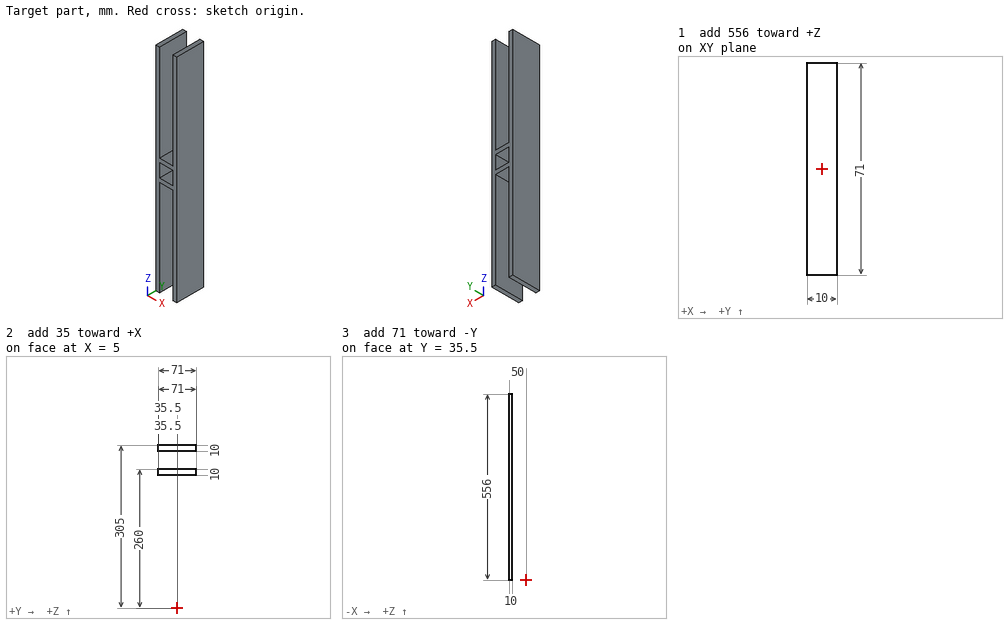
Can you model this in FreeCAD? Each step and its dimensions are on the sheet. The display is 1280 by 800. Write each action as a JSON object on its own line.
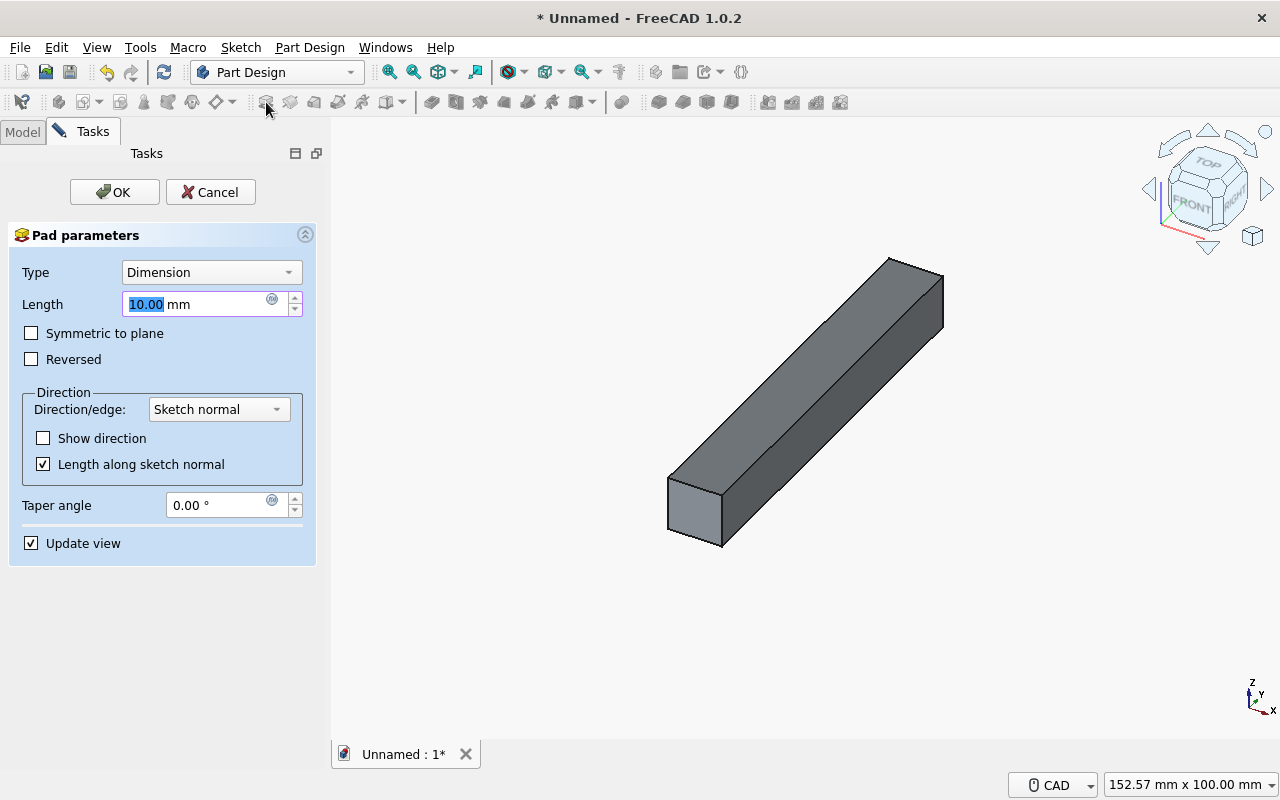
{"action": "type", "text": "556"}
{"action": "key", "text": "Tab"}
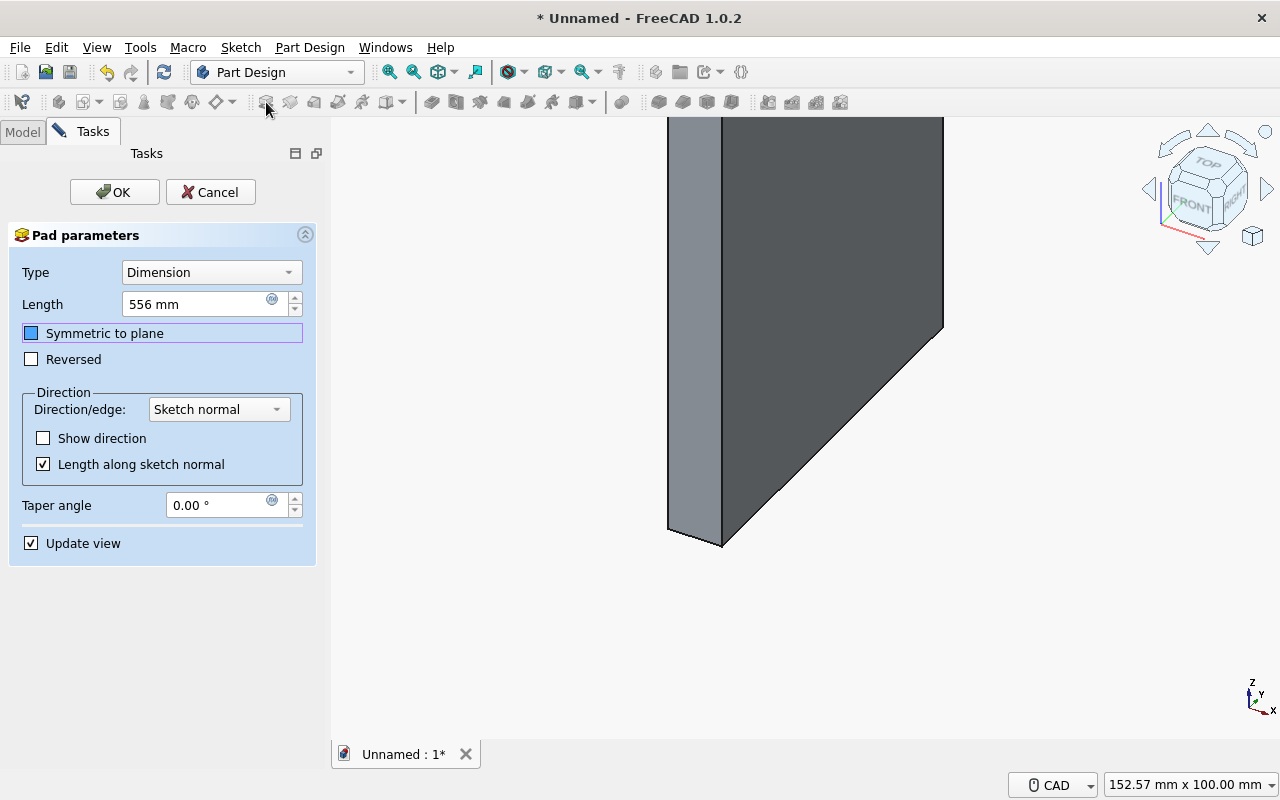
{"action": "left_click", "coordinate": [115, 192]}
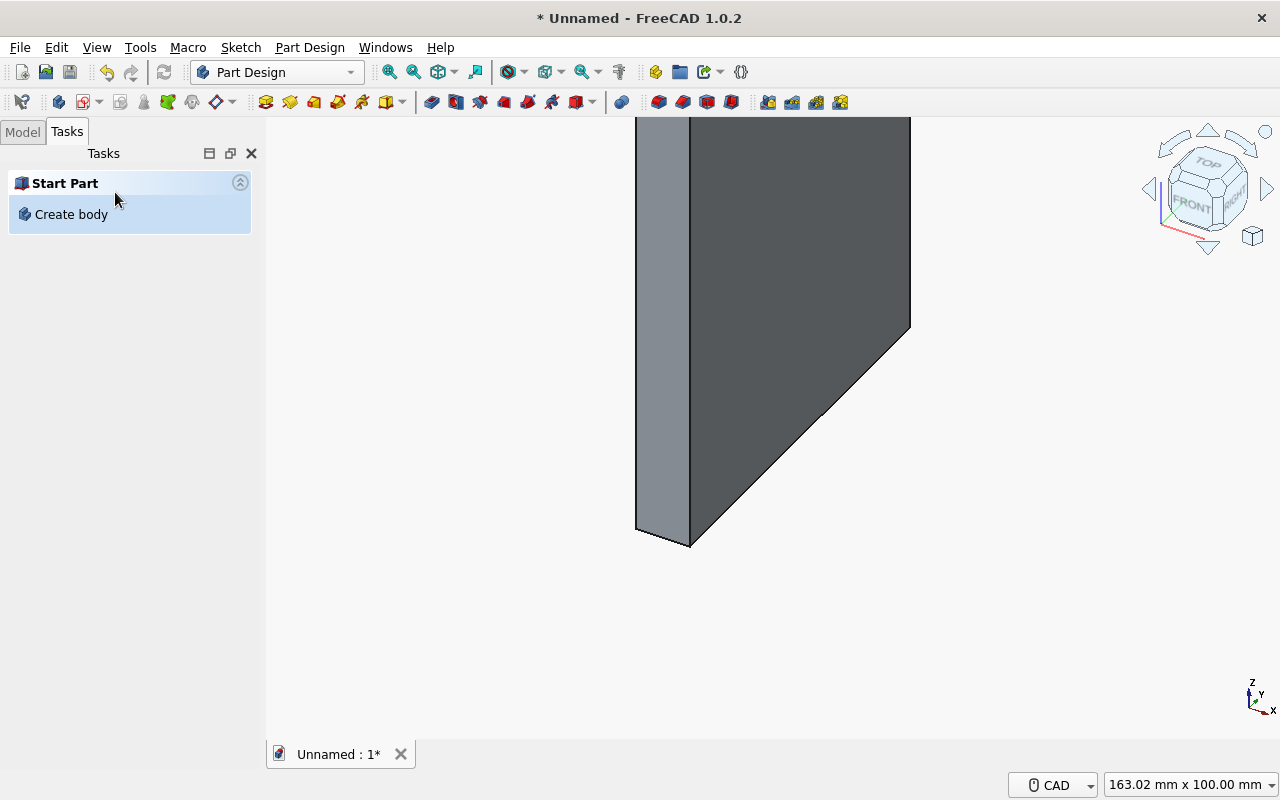
{"action": "left_click", "coordinate": [390, 72]}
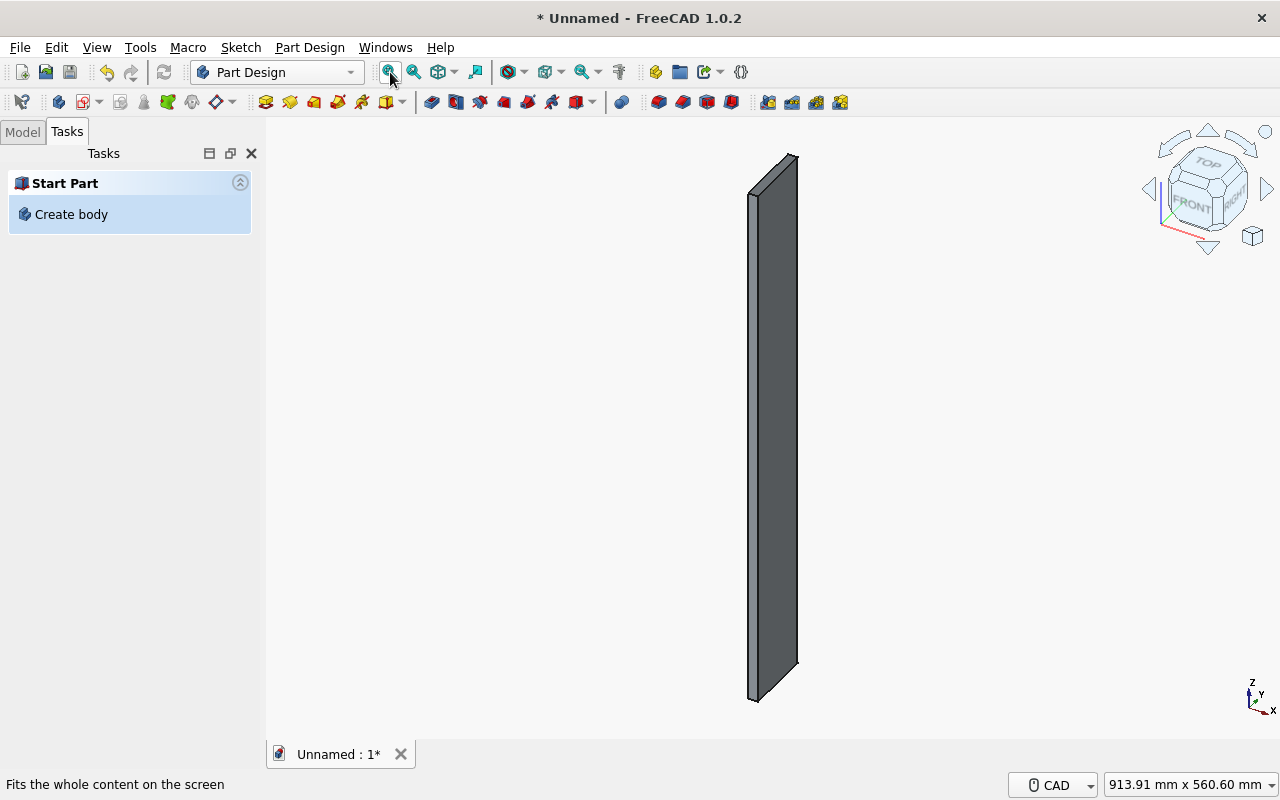
{"action": "left_click", "coordinate": [778, 212]}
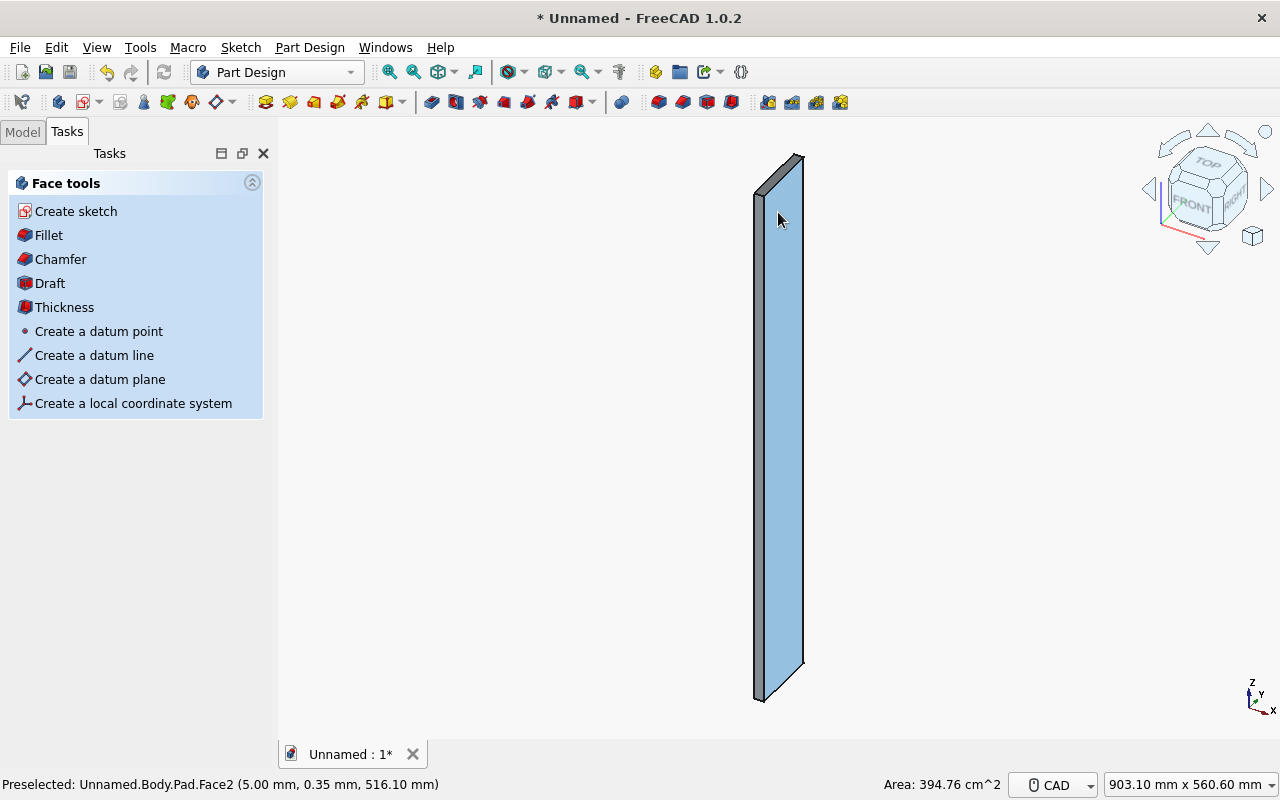
{"action": "left_click", "coordinate": [84, 102]}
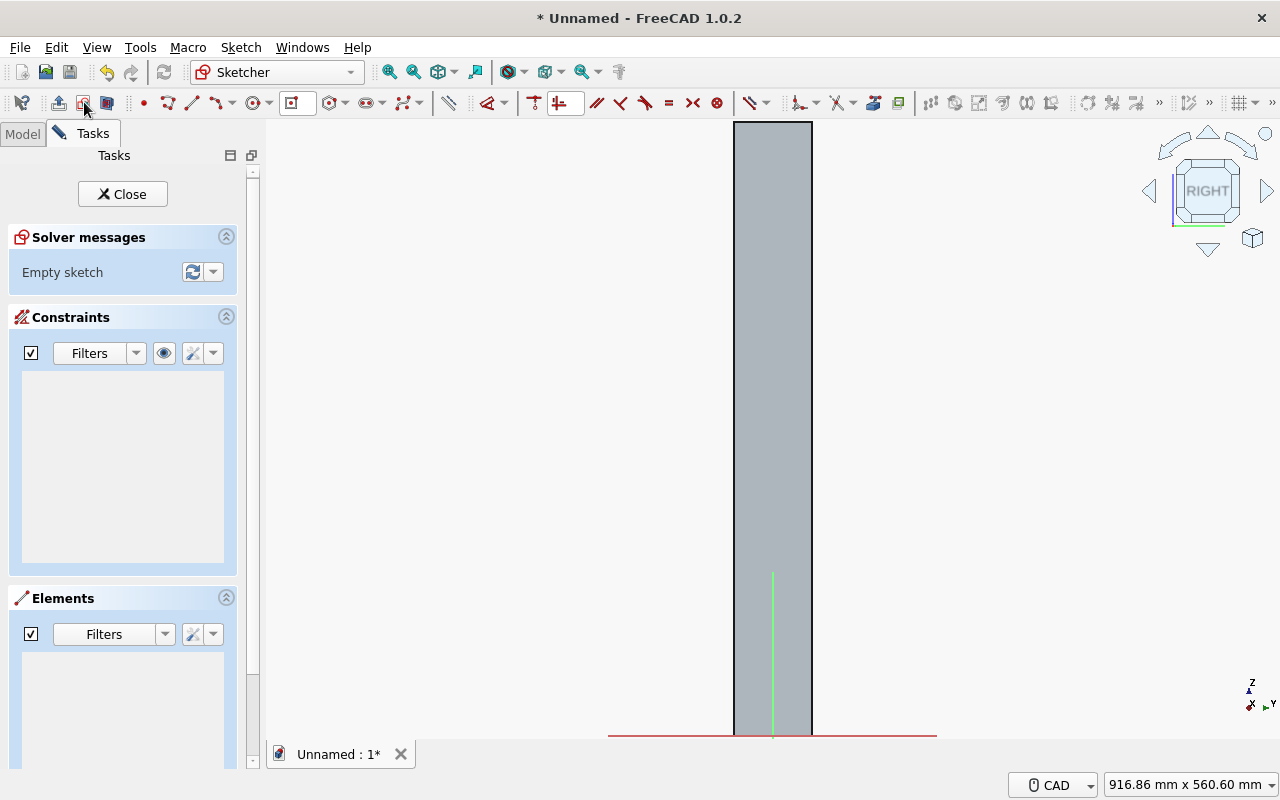
{"action": "scroll", "coordinate": [787, 430], "scroll_direction": "up", "scroll_amount": 9}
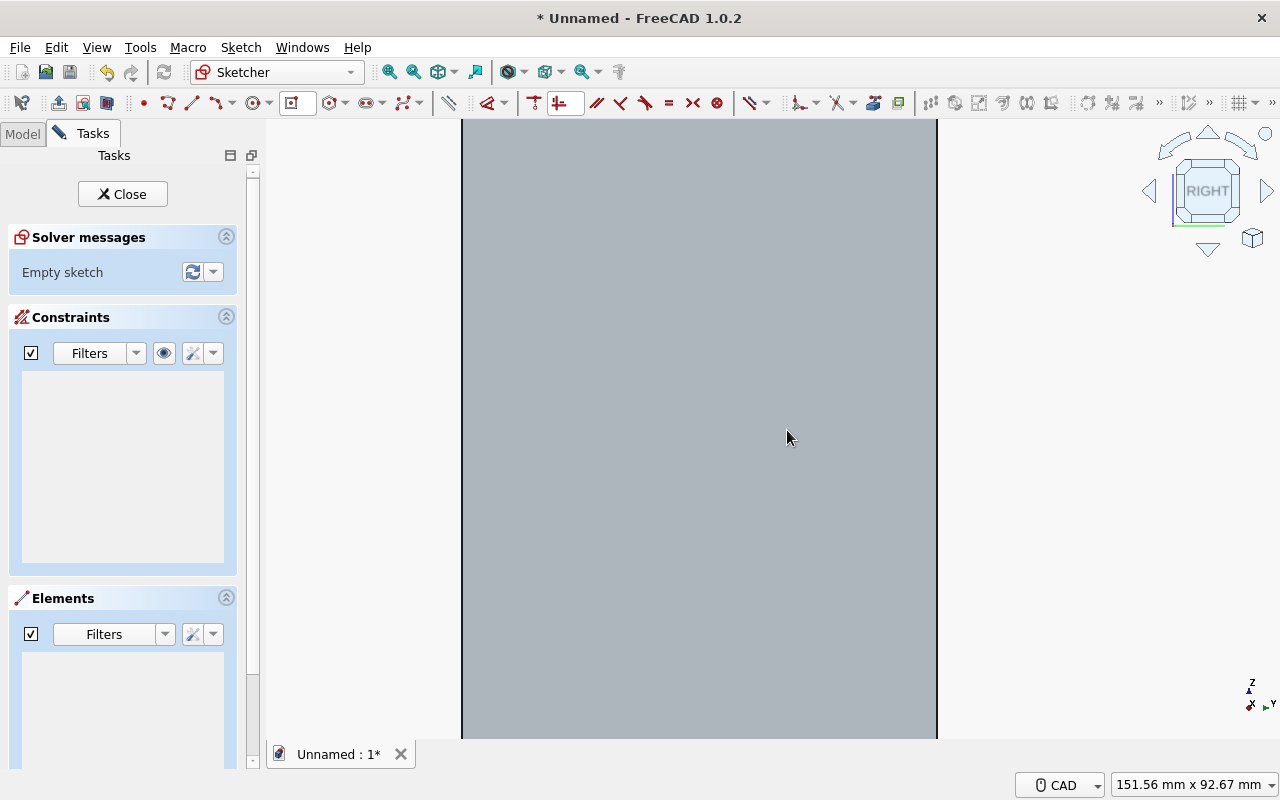
{"action": "key", "text": "g r"}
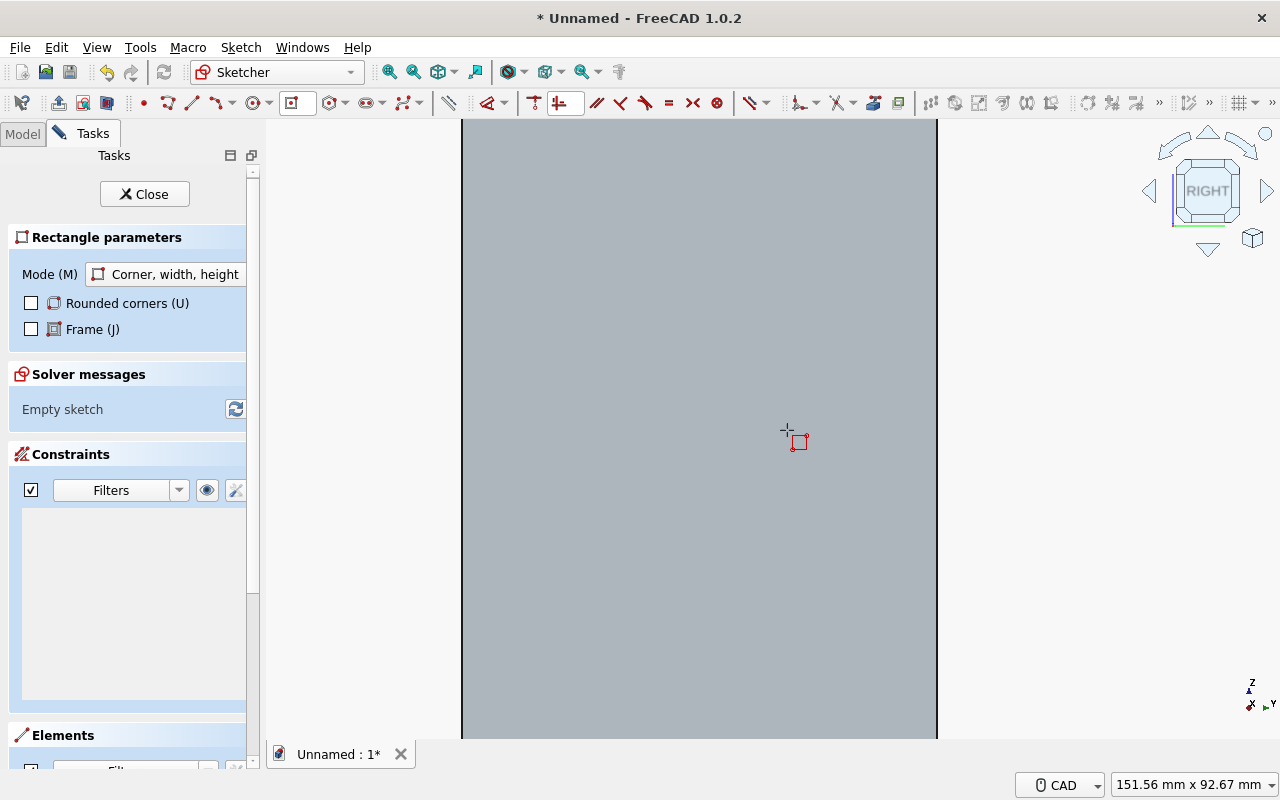
{"action": "left_click", "coordinate": [462, 241]}
{"action": "mouse_move", "coordinate": [937, 308]}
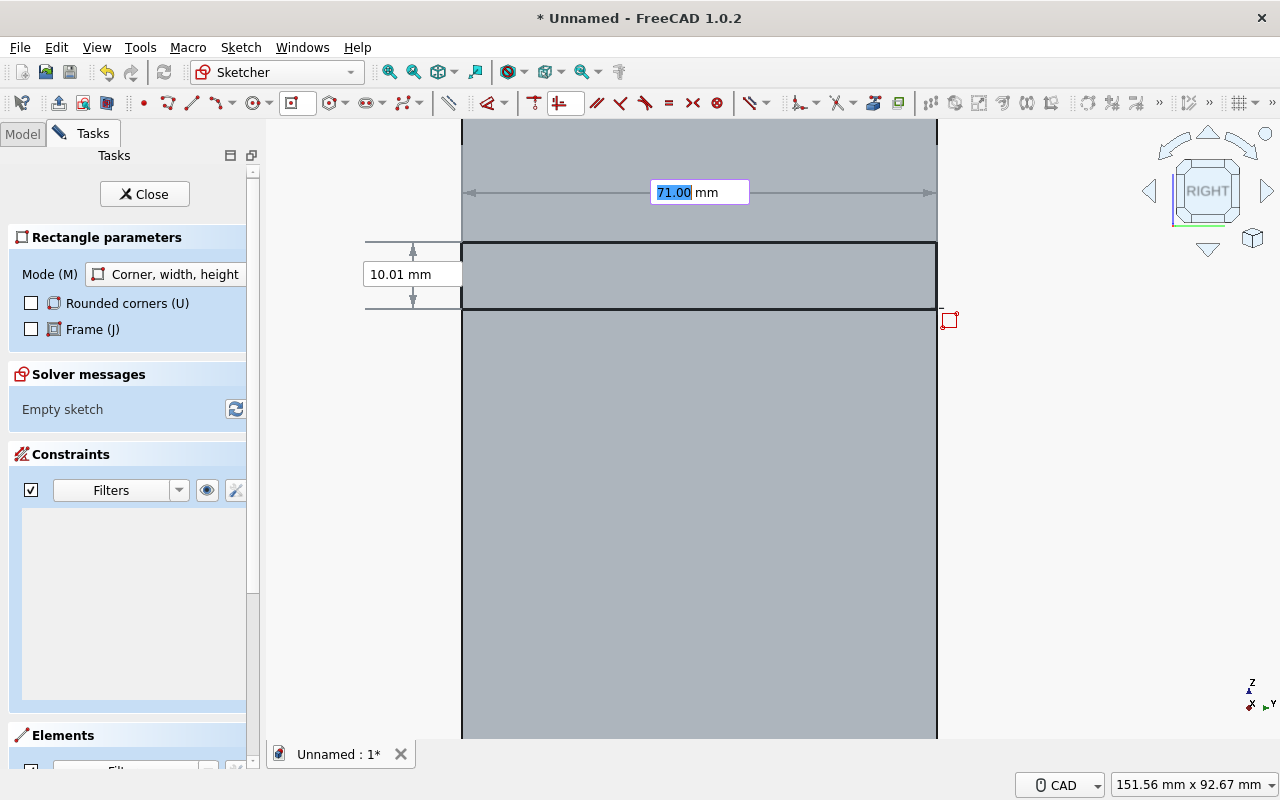
{"action": "type", "text": "71"}
{"action": "key", "text": "Tab"}
{"action": "type", "text": "10"}
{"action": "key", "text": "Return"}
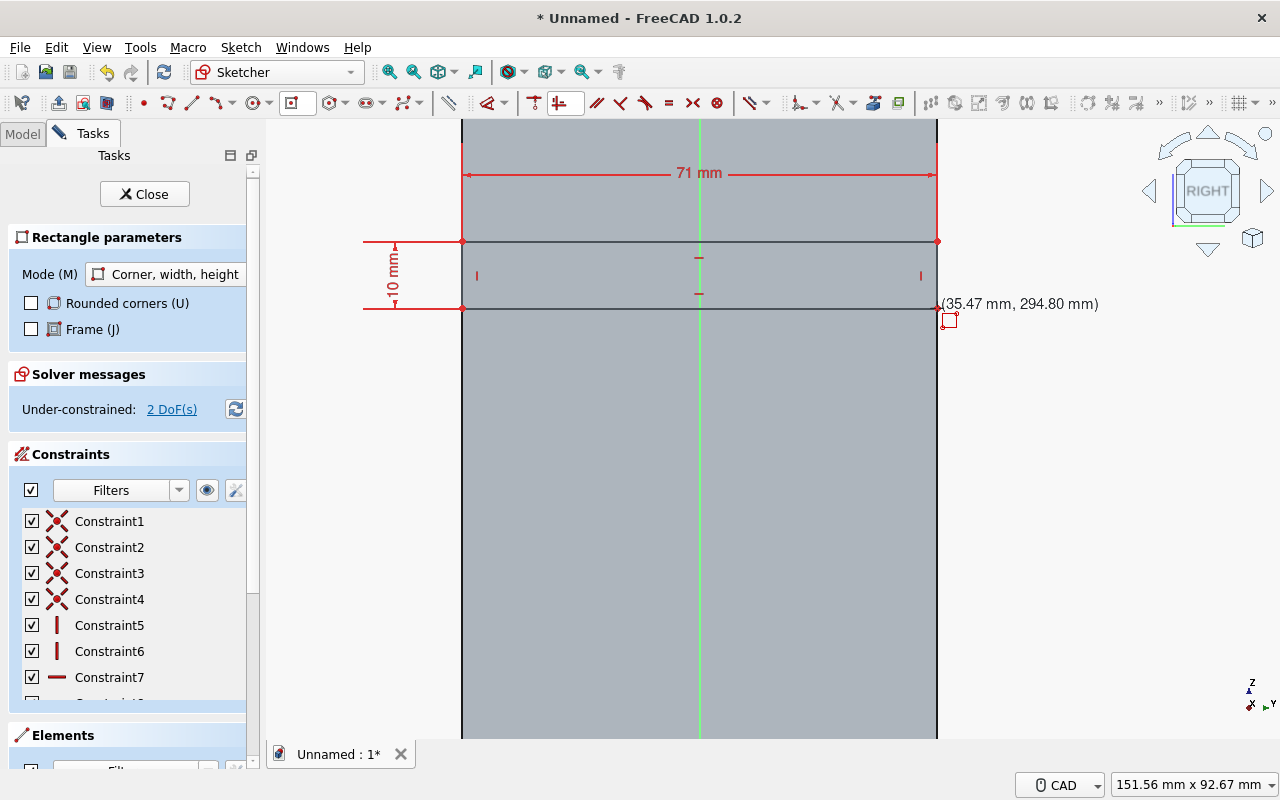
{"action": "left_click", "coordinate": [462, 542]}
{"action": "mouse_move", "coordinate": [937, 609]}